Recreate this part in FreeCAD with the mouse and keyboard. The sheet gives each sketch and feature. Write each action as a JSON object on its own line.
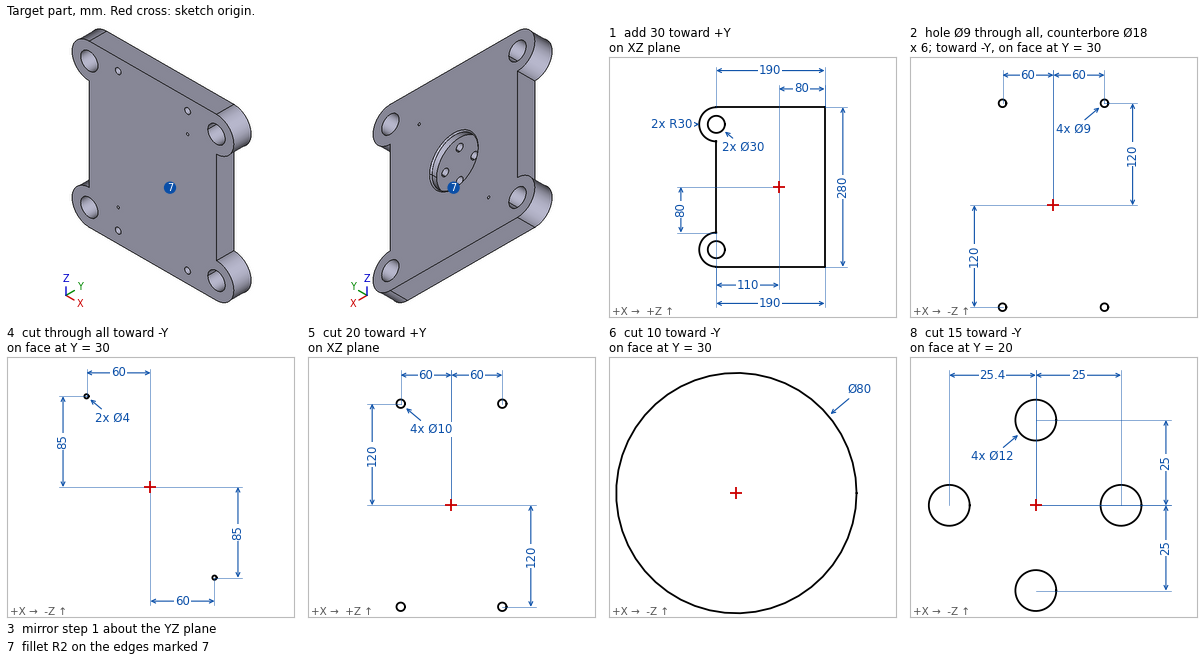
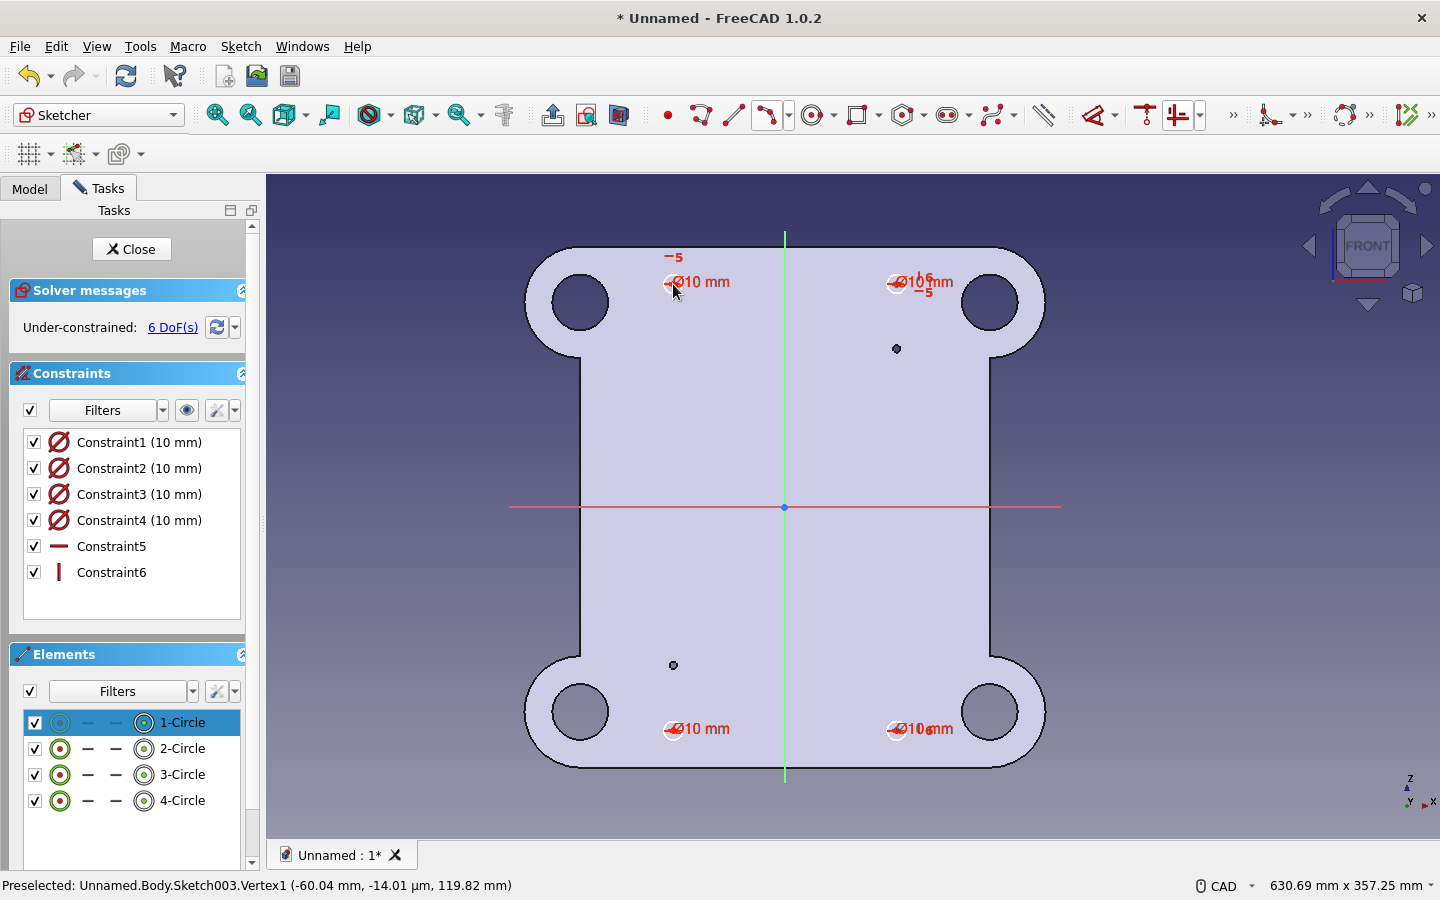
{"action": "left_click", "coordinate": [673, 731]}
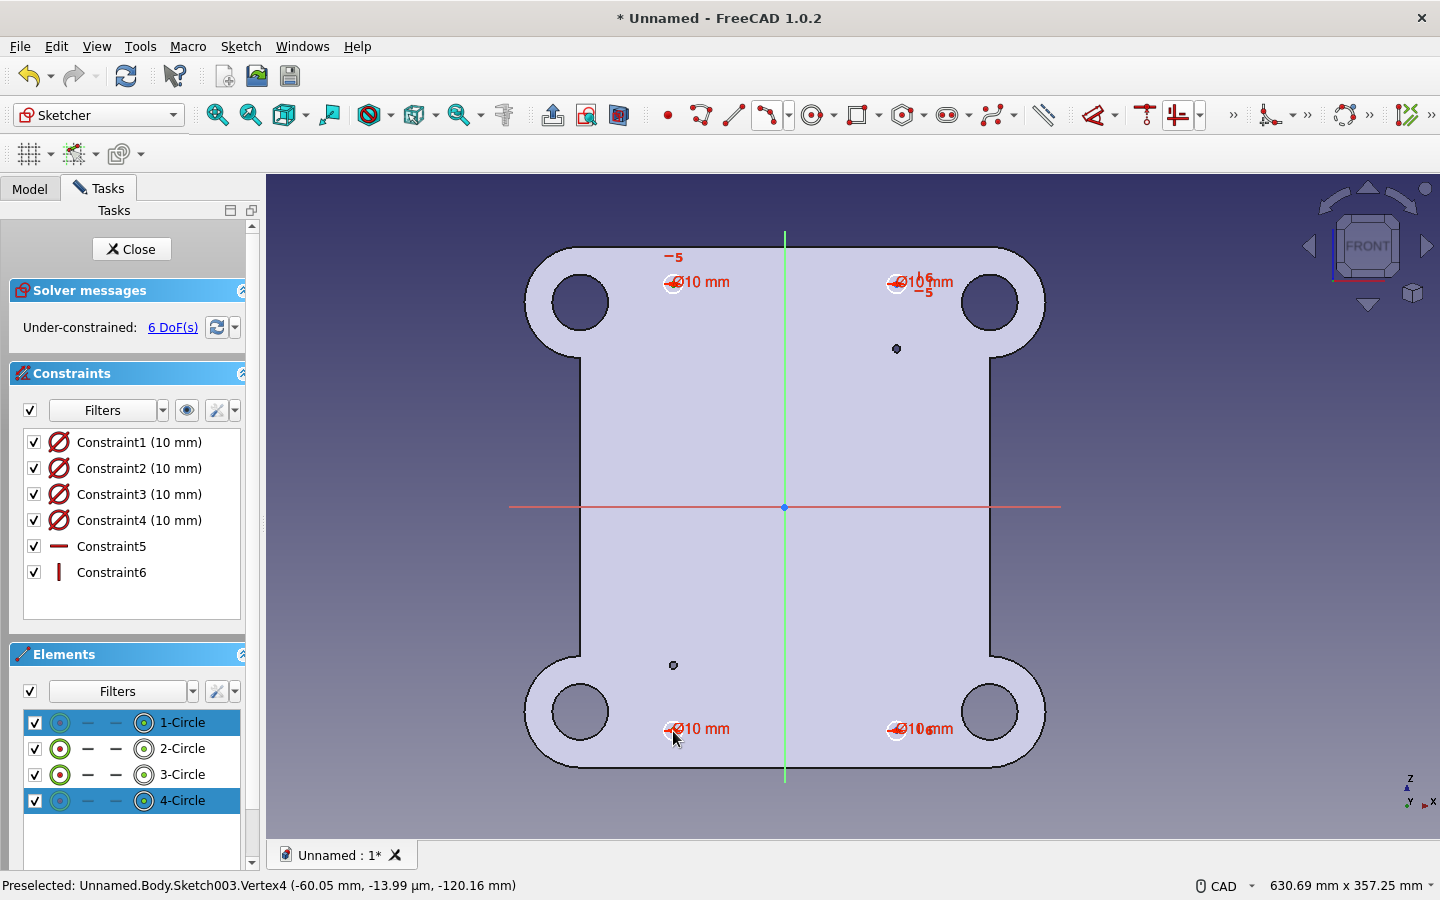
{"action": "key", "text": "v"}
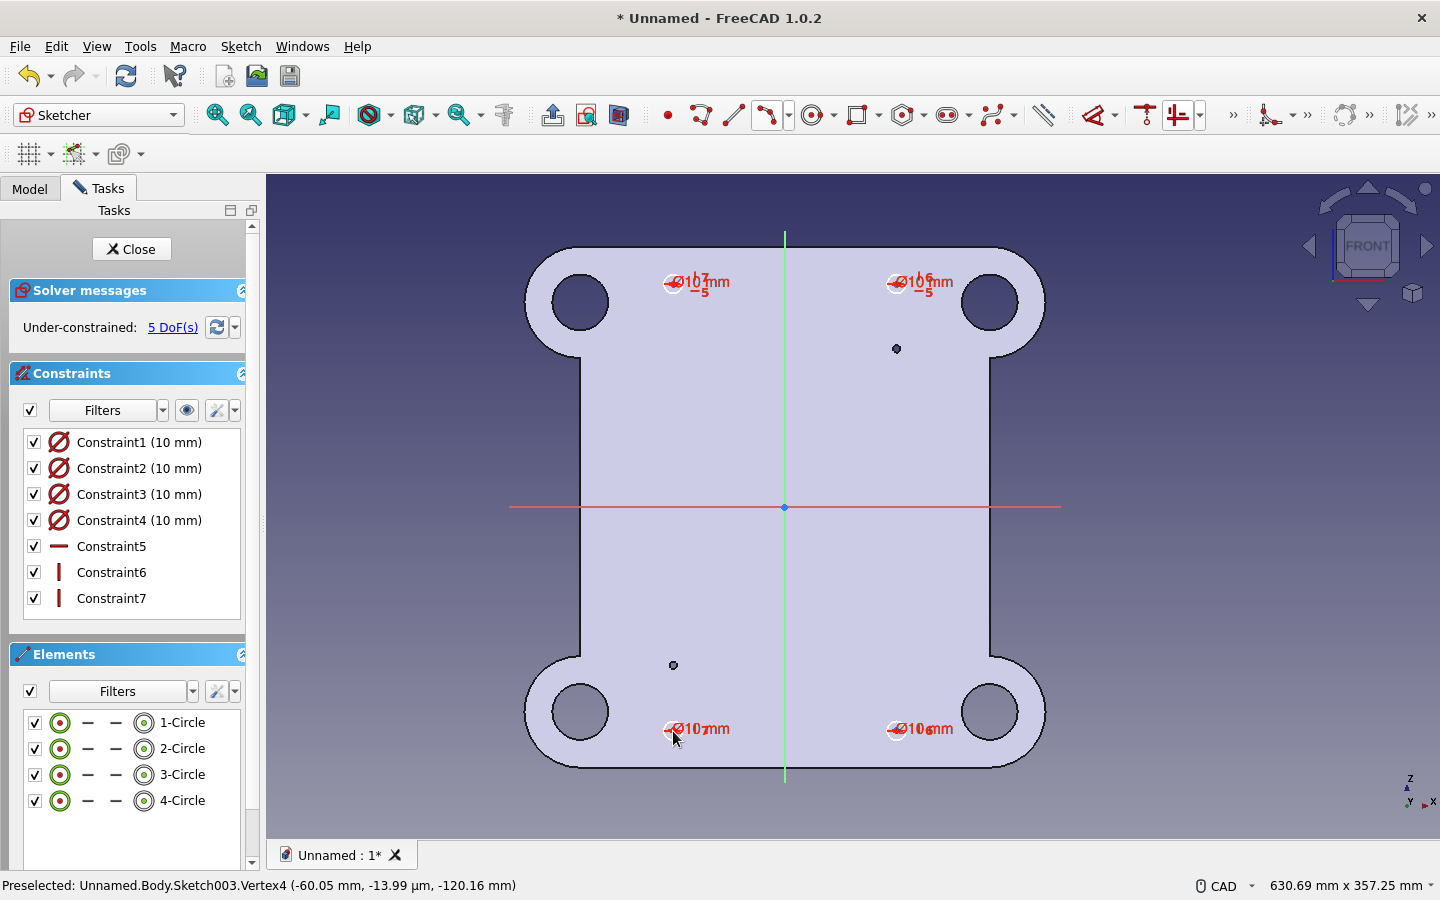
{"action": "left_click", "coordinate": [897, 731]}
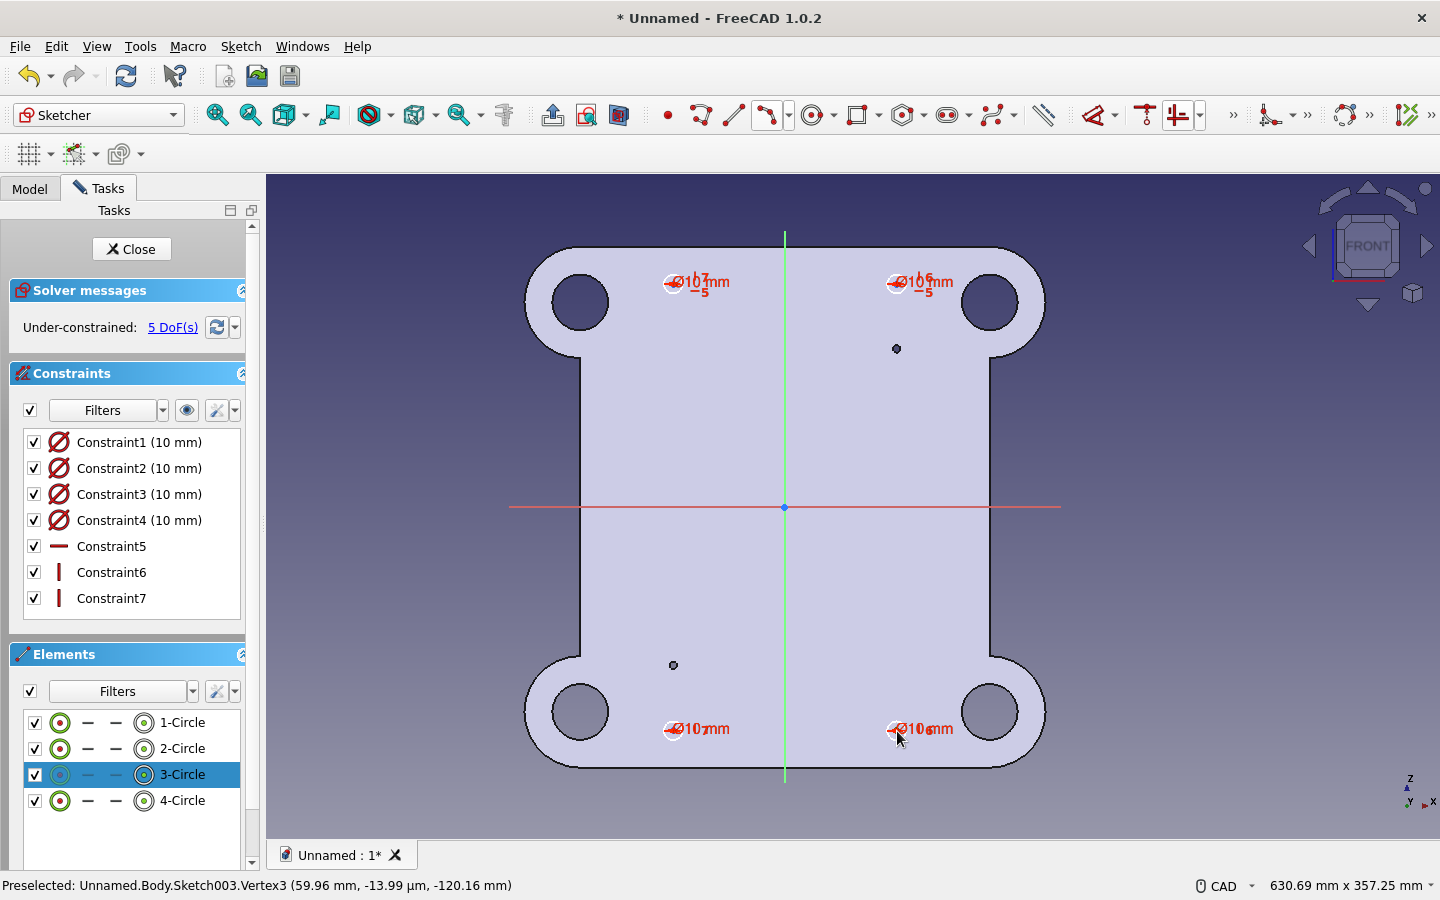
{"action": "left_click", "coordinate": [673, 731]}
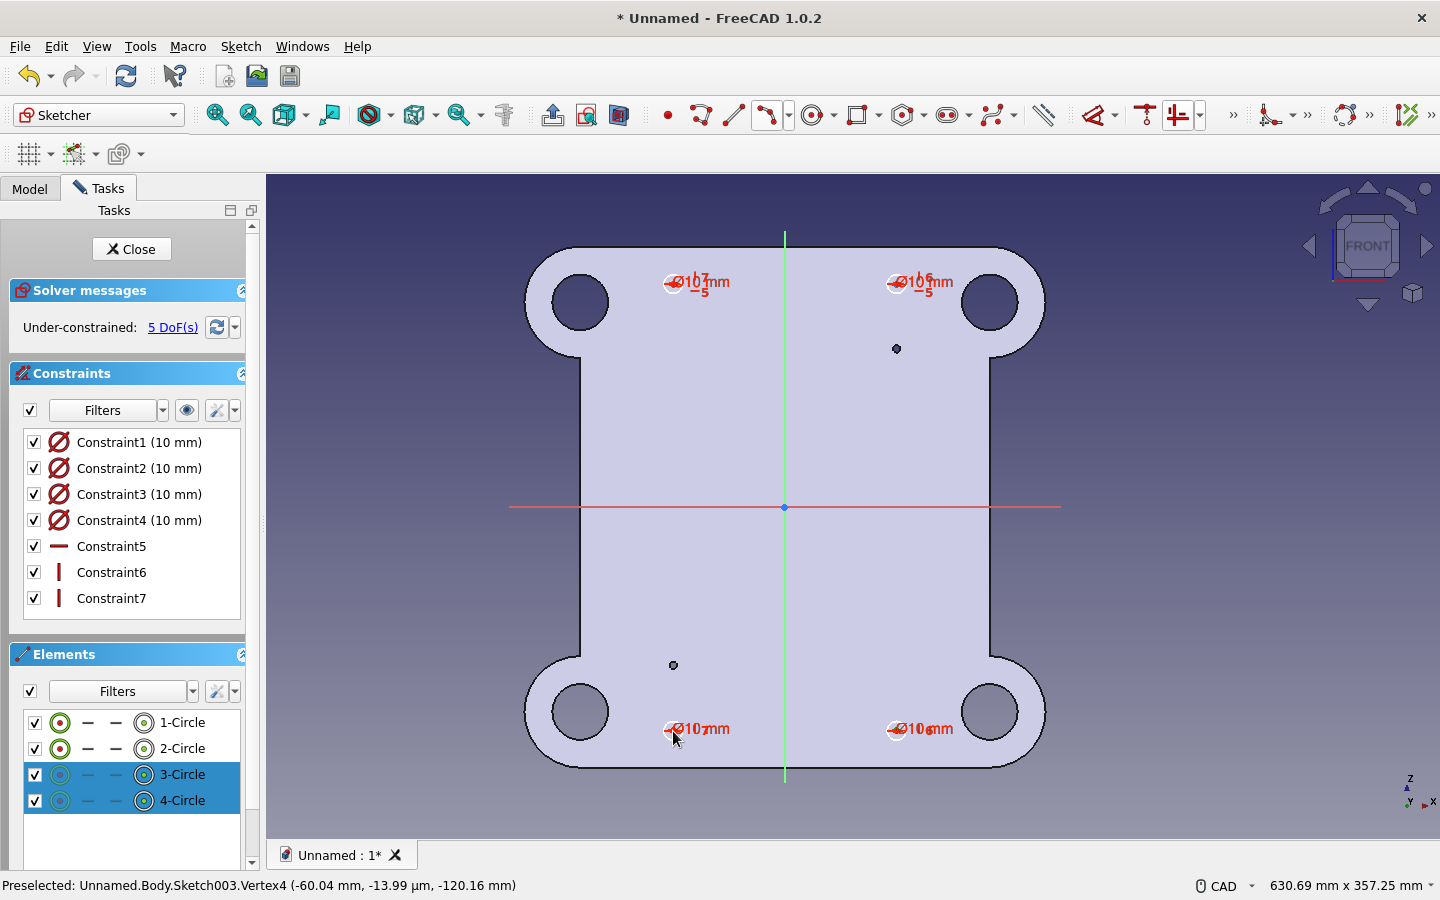
{"action": "left_click", "coordinate": [1200, 116]}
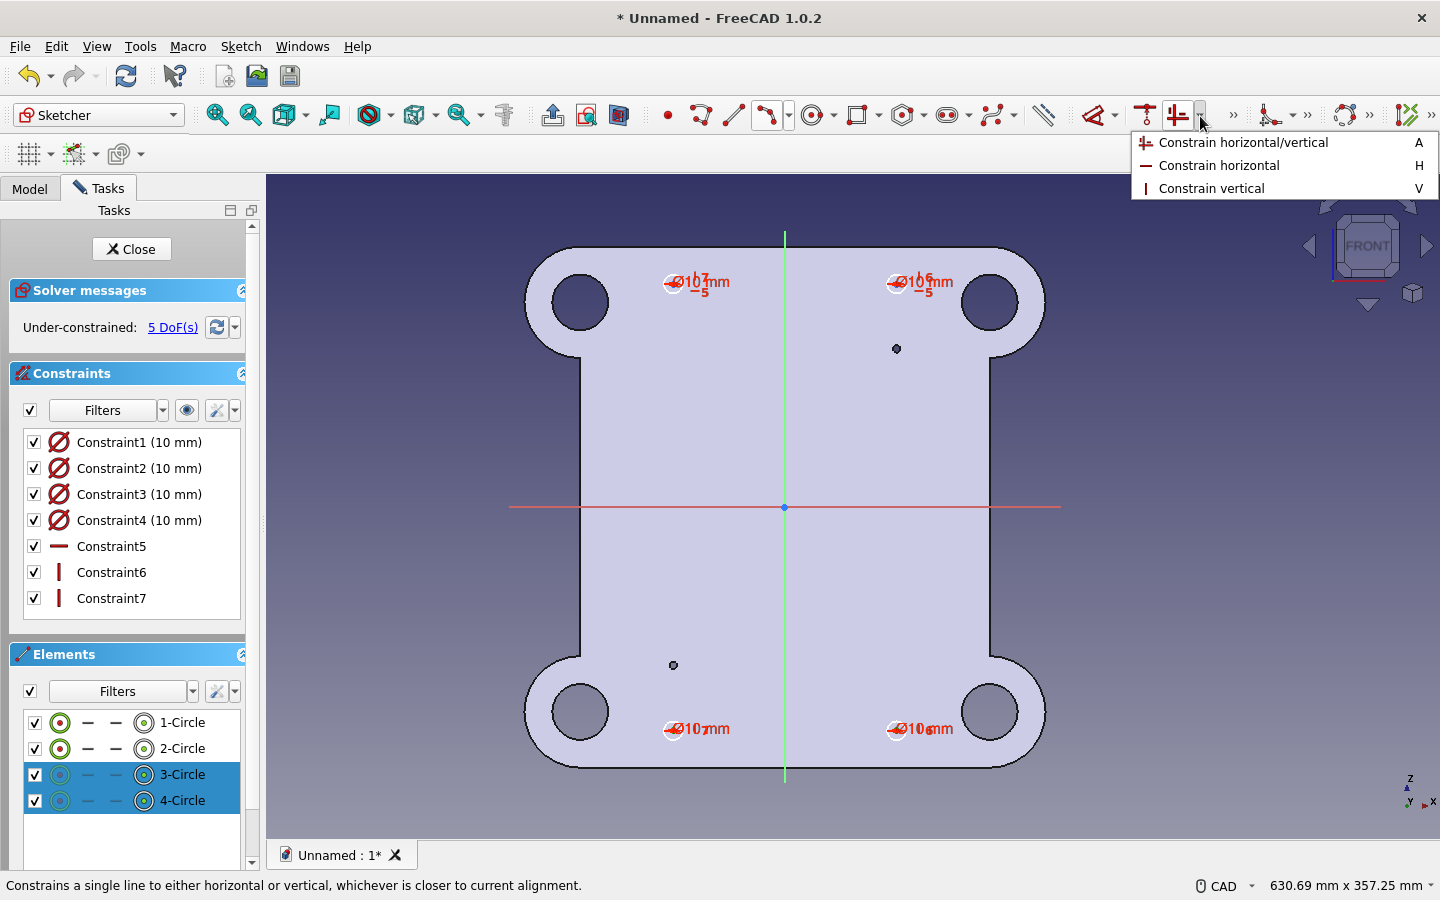
{"action": "left_click", "coordinate": [1285, 166]}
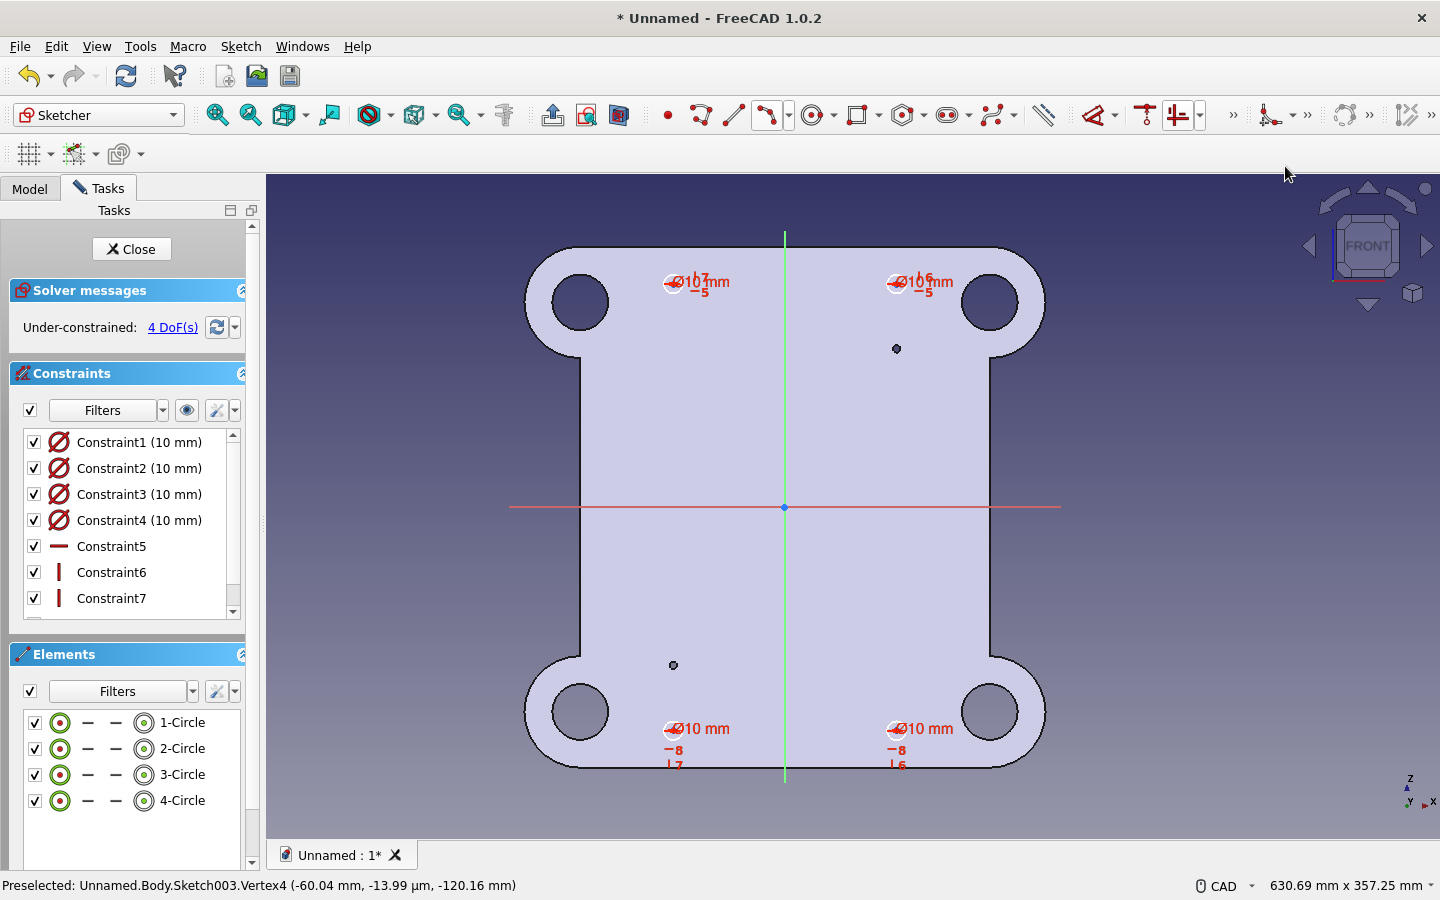
{"action": "left_click", "coordinate": [1092, 116]}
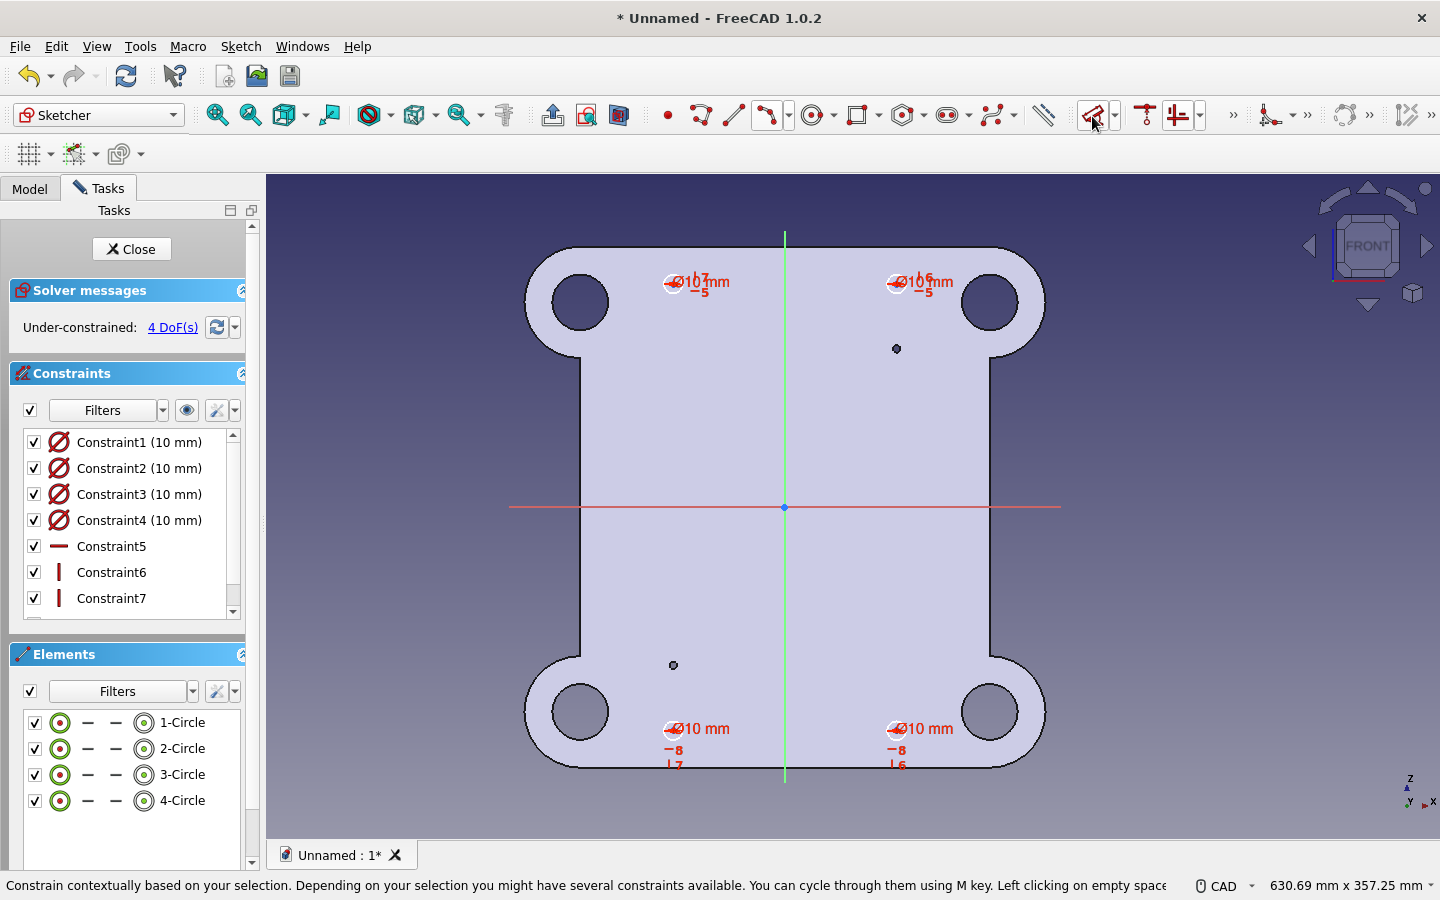
{"action": "left_click", "coordinate": [673, 284]}
{"action": "left_click", "coordinate": [729, 250]}